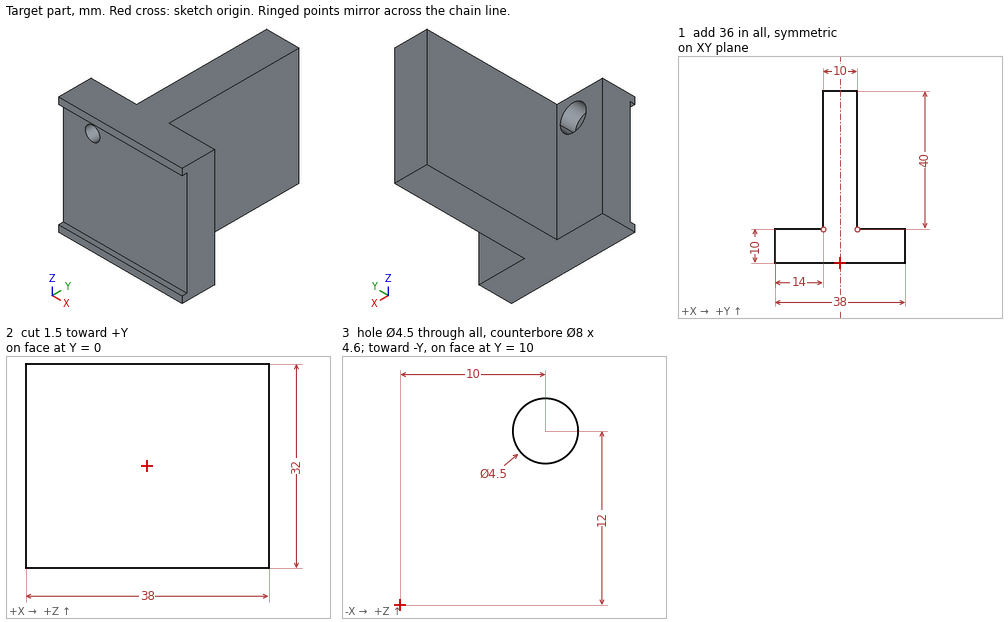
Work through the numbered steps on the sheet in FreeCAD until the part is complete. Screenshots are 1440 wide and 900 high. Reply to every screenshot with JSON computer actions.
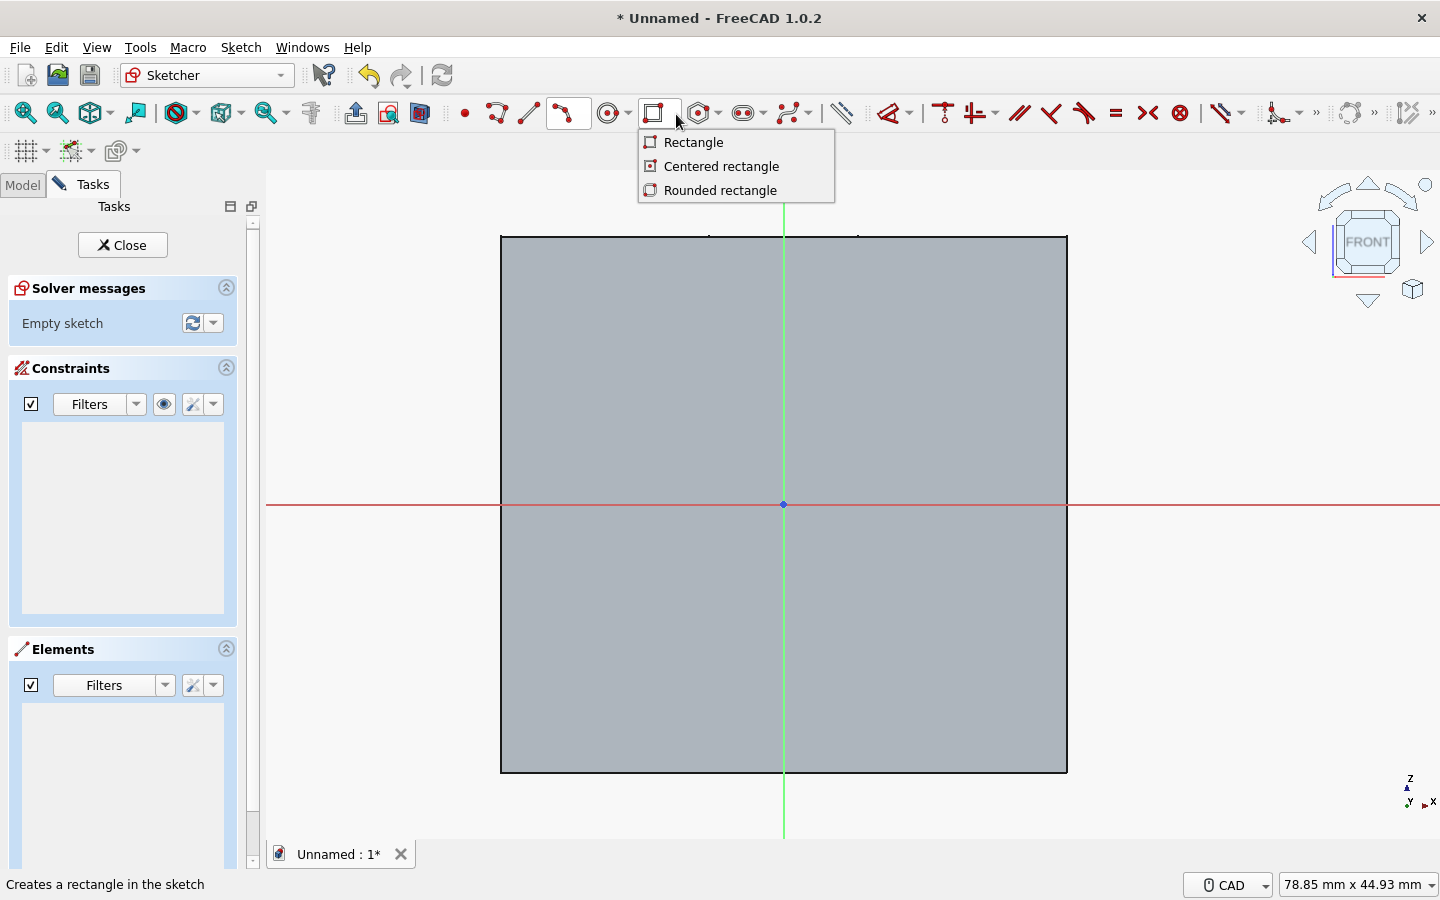
{"action": "left_click", "coordinate": [736, 166]}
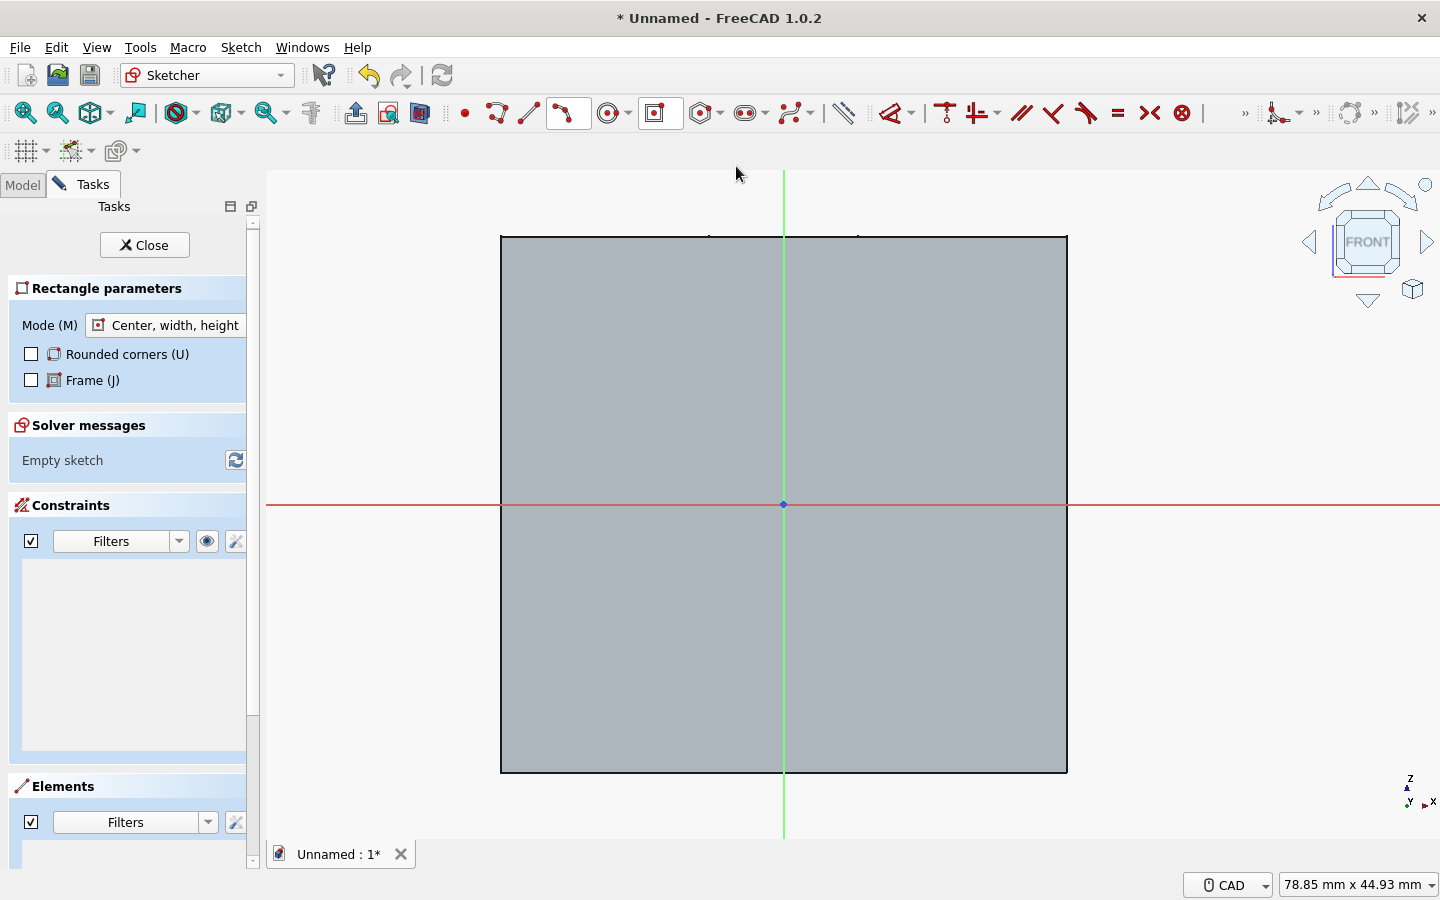
{"action": "left_click", "coordinate": [784, 504]}
{"action": "left_click", "coordinate": [1067, 266]}
{"action": "key", "text": "Escape"}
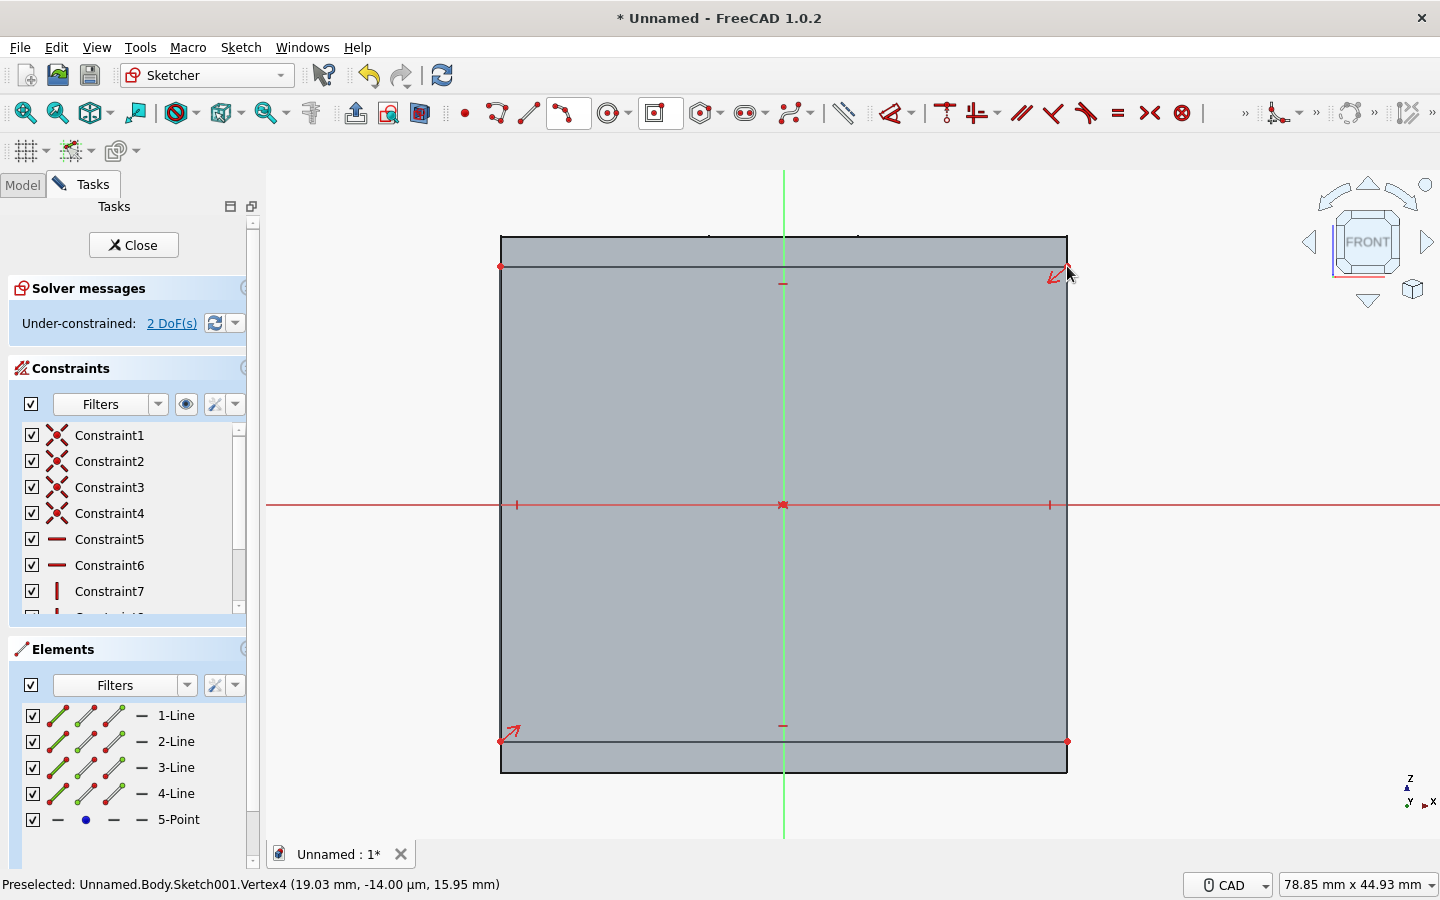
{"action": "left_click", "coordinate": [890, 114]}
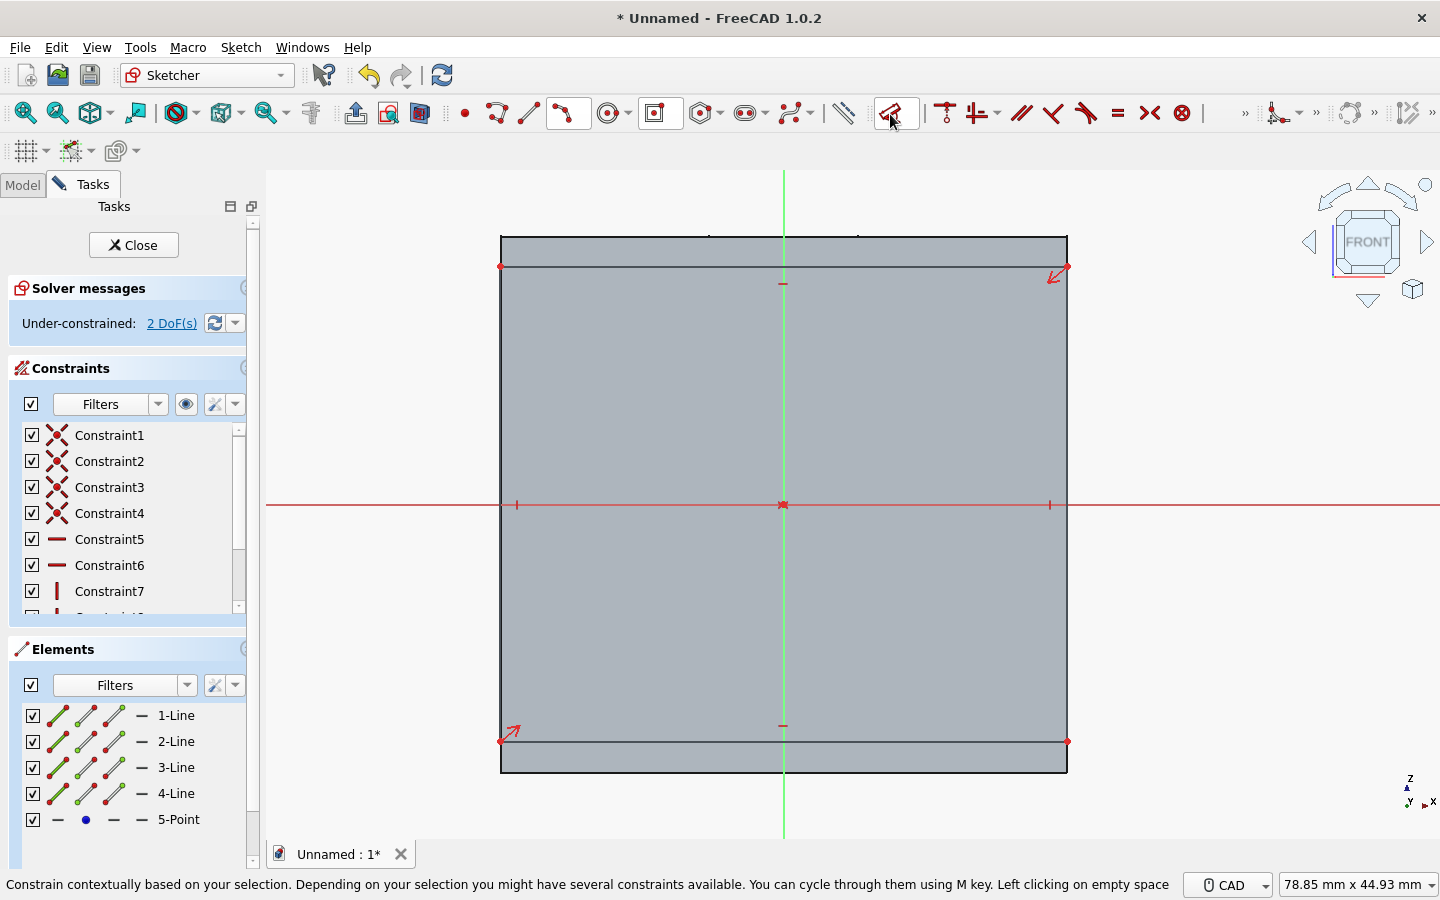
{"action": "left_click", "coordinate": [670, 742]}
{"action": "left_click", "coordinate": [653, 776]}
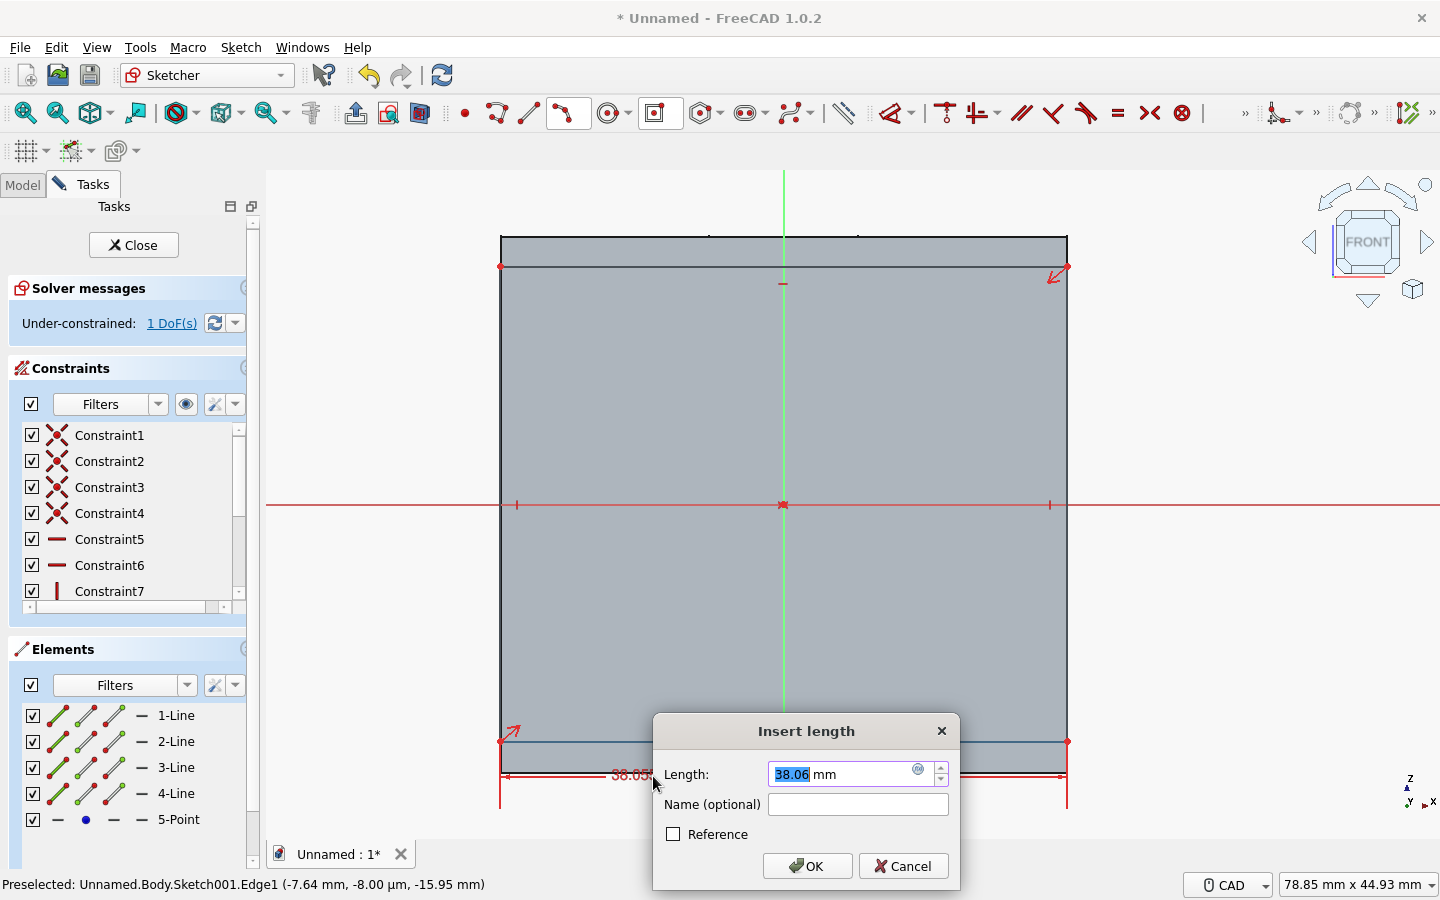
{"action": "type", "text": "38"}
{"action": "key", "text": "Return"}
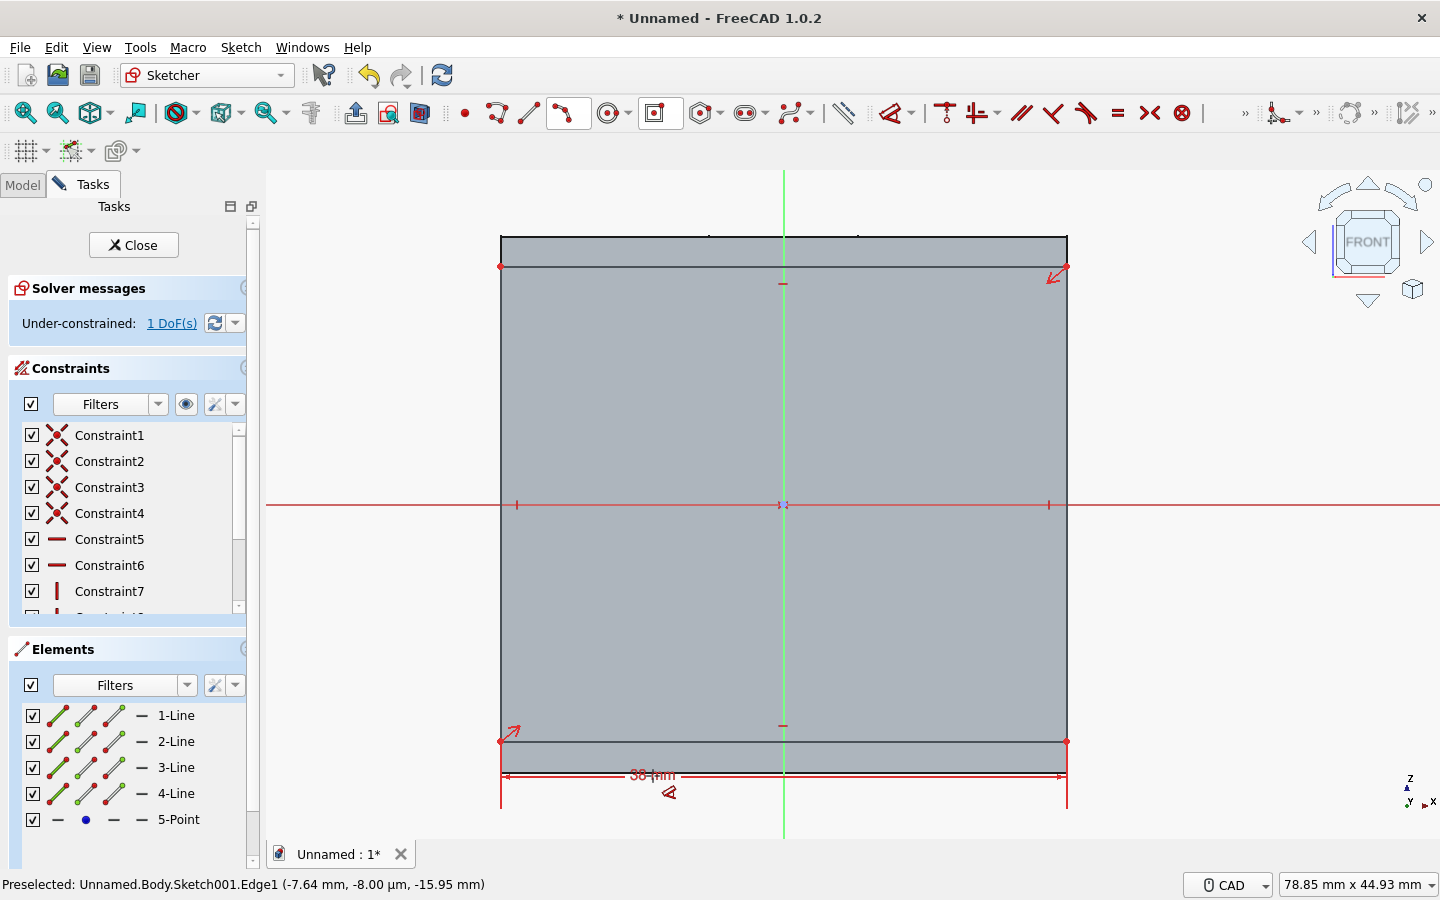
{"action": "left_click", "coordinate": [1067, 599]}
{"action": "left_click", "coordinate": [1101, 395]}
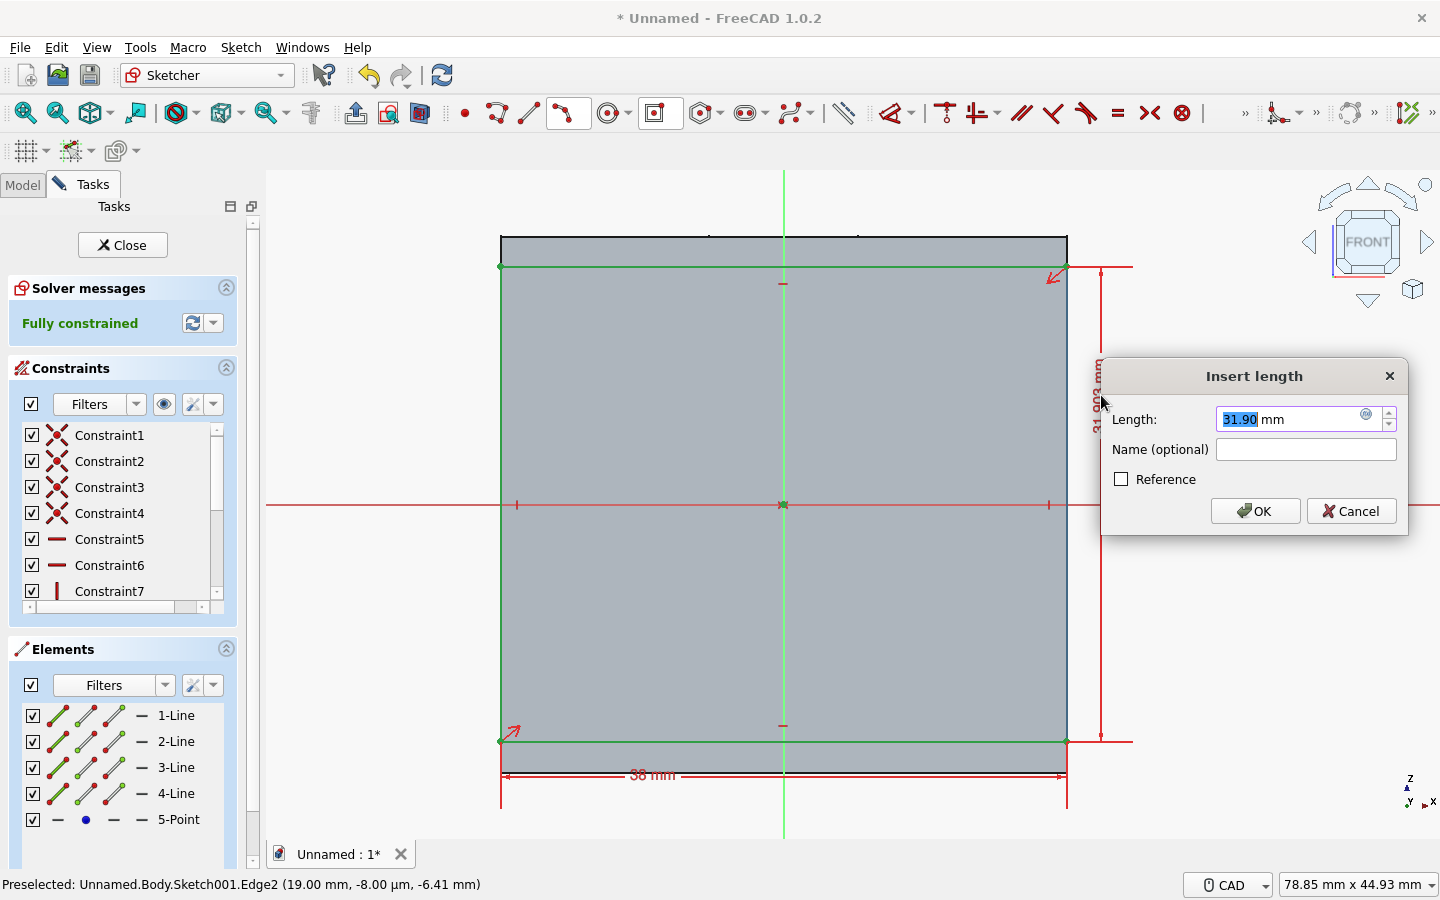
{"action": "type", "text": "32"}
{"action": "key", "text": "Return"}
{"action": "key", "text": "Escape"}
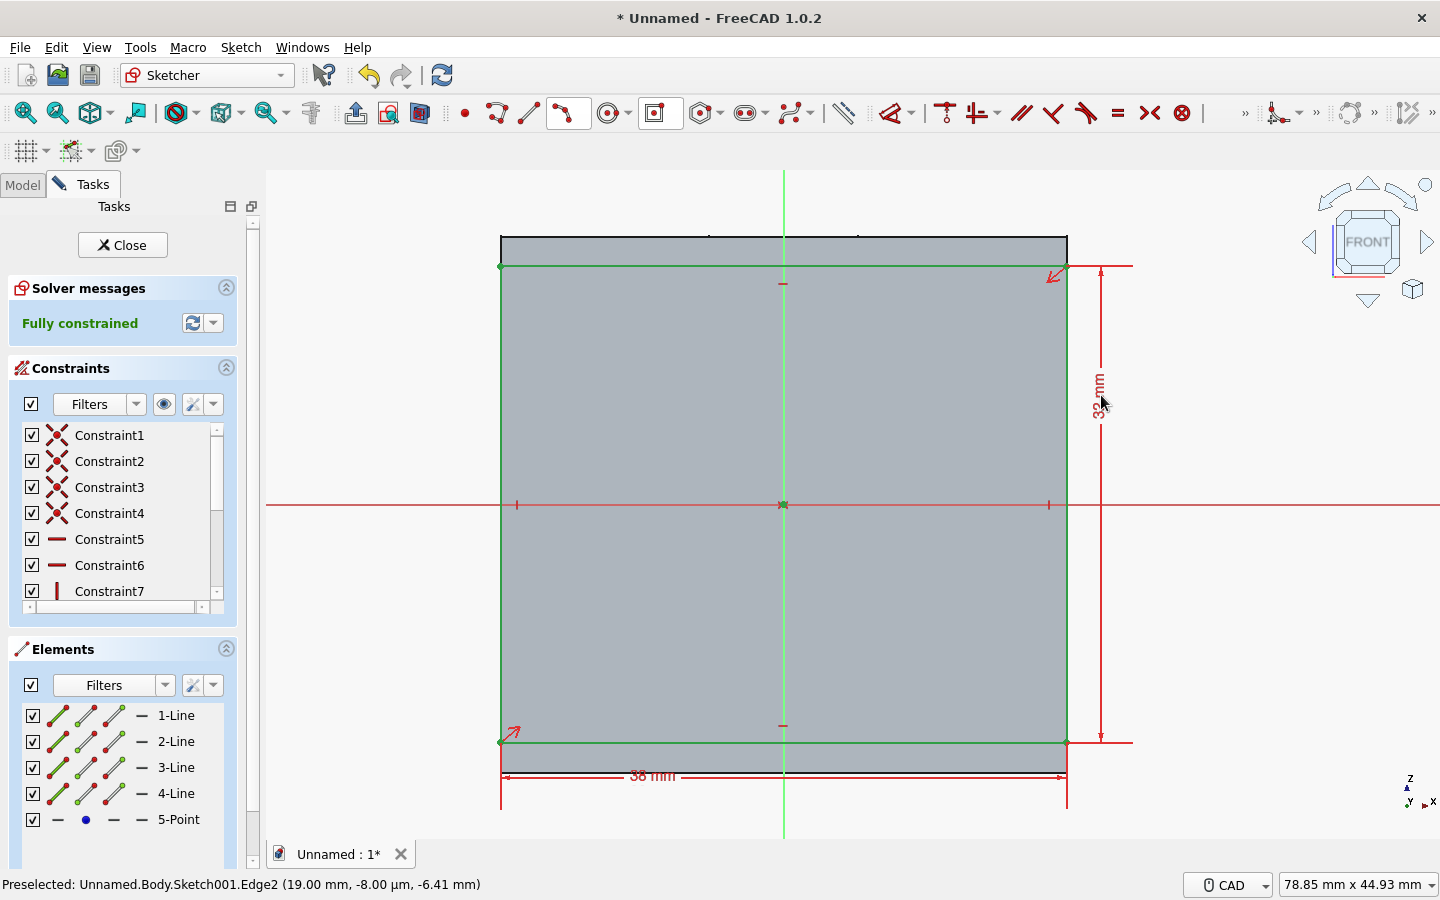
{"action": "left_click", "coordinate": [123, 245]}